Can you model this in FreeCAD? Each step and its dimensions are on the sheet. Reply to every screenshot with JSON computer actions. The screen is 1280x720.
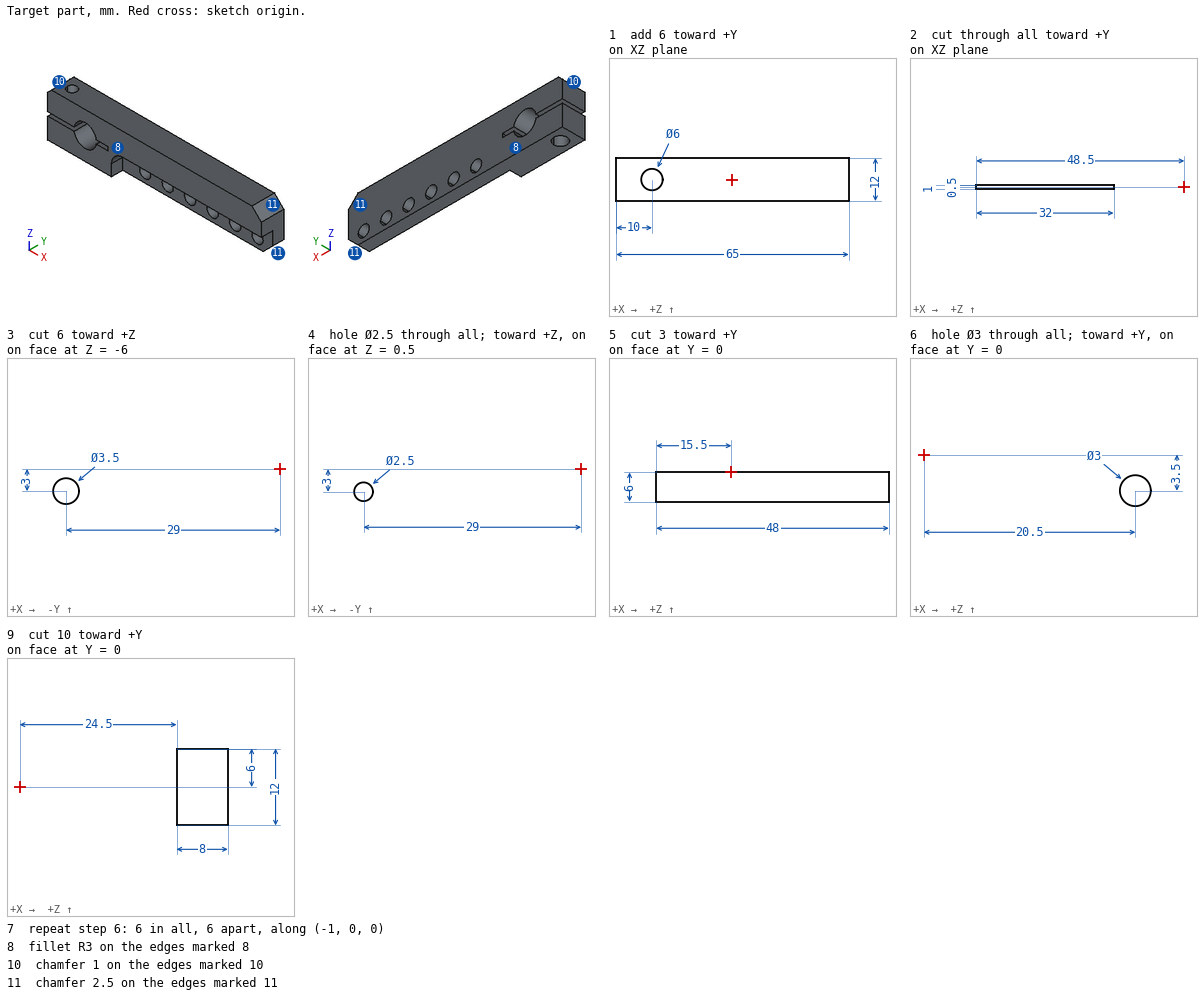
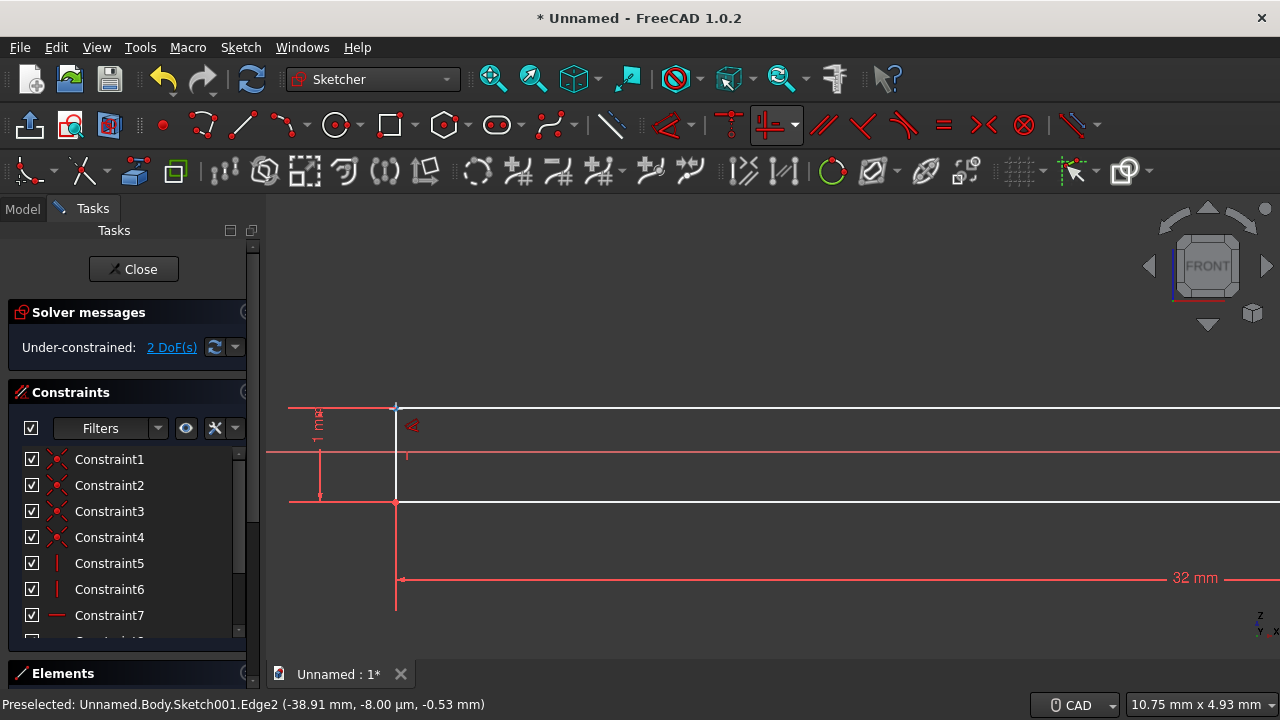
{"action": "left_click", "coordinate": [396, 408]}
{"action": "left_click", "coordinate": [362, 430]}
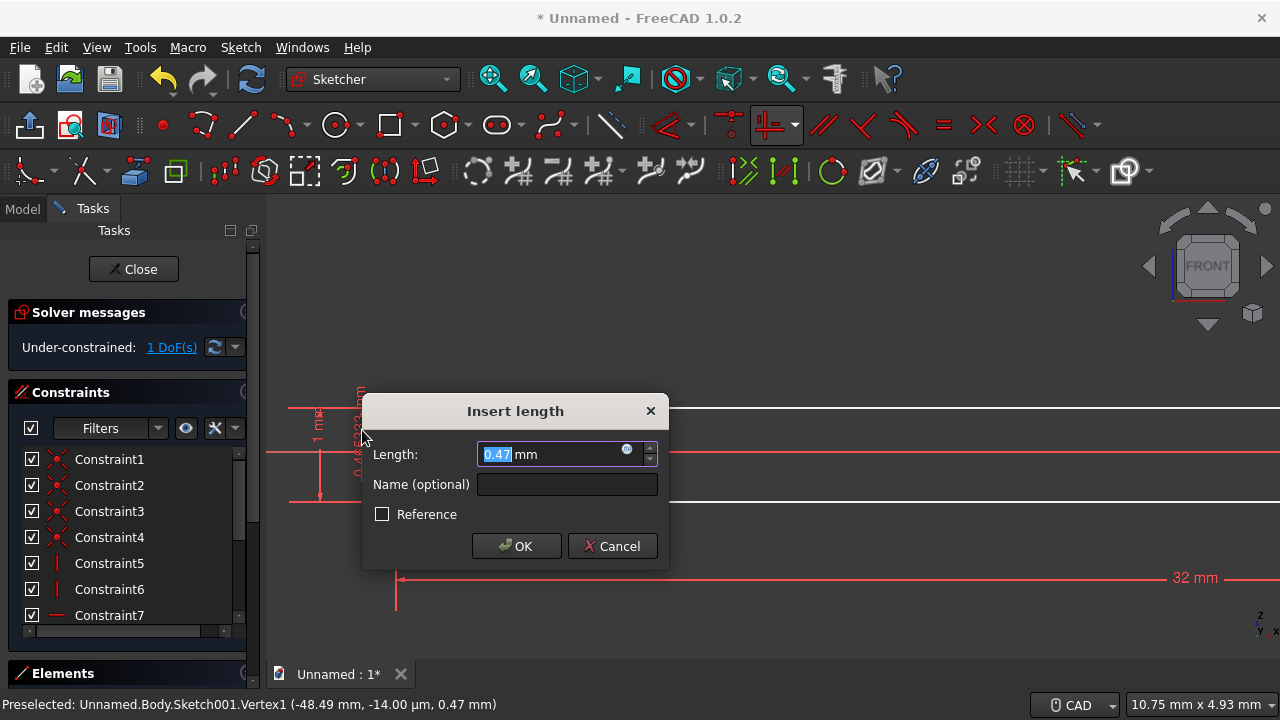
{"action": "type", "text": "0.5"}
{"action": "key", "text": "Return"}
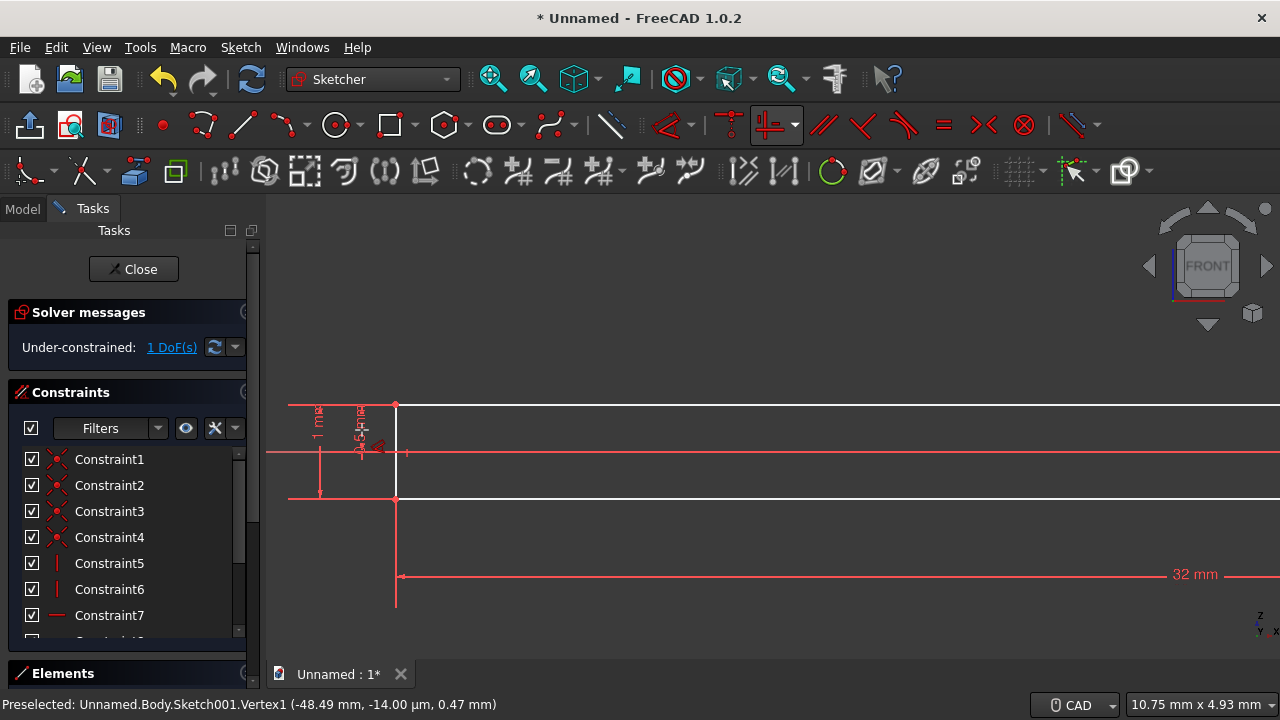
{"action": "scroll", "coordinate": [395, 422], "scroll_direction": "down", "scroll_amount": 10}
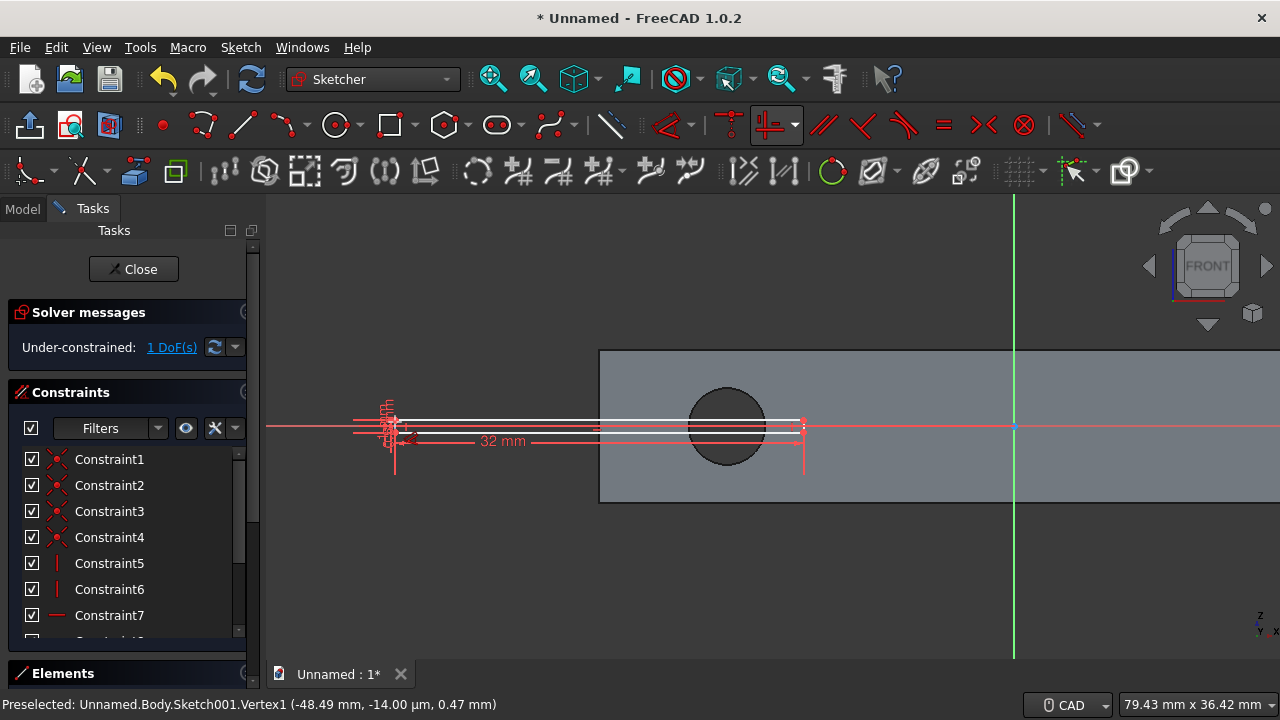
{"action": "left_click", "coordinate": [395, 420]}
{"action": "left_click", "coordinate": [705, 386]}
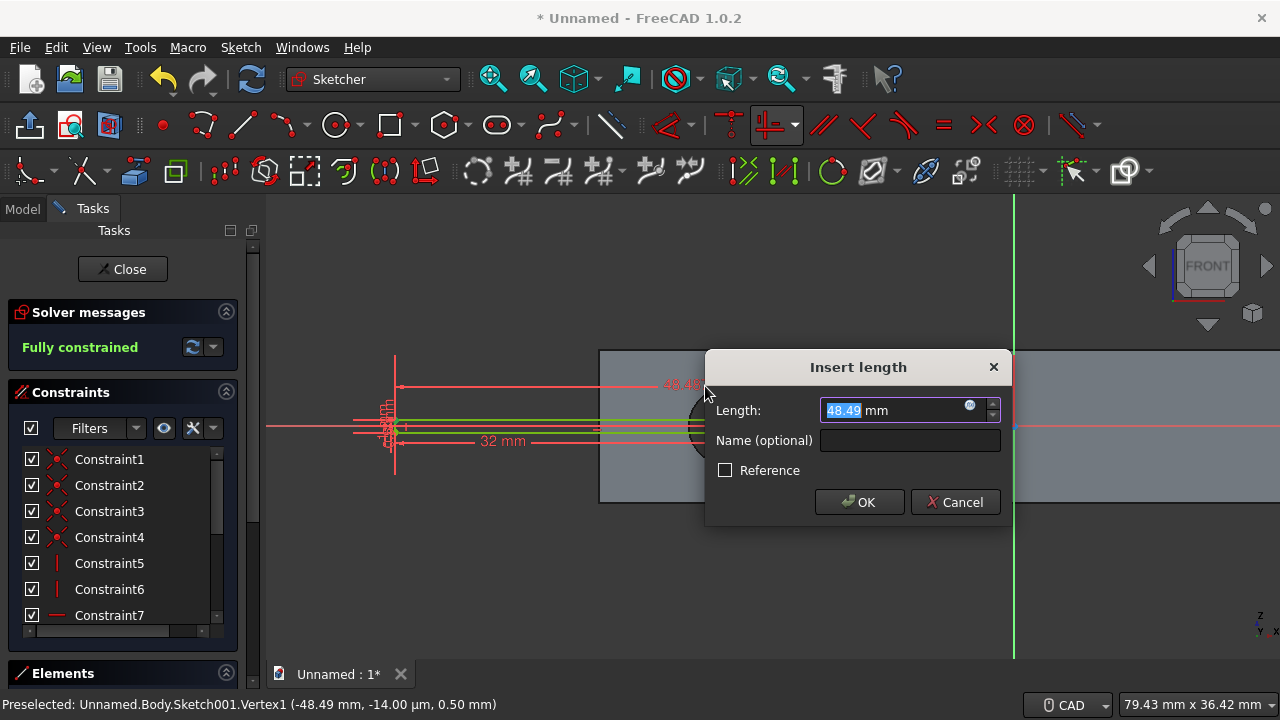
{"action": "type", "text": "48.5"}
{"action": "key", "text": "Return"}
{"action": "key", "text": "Escape"}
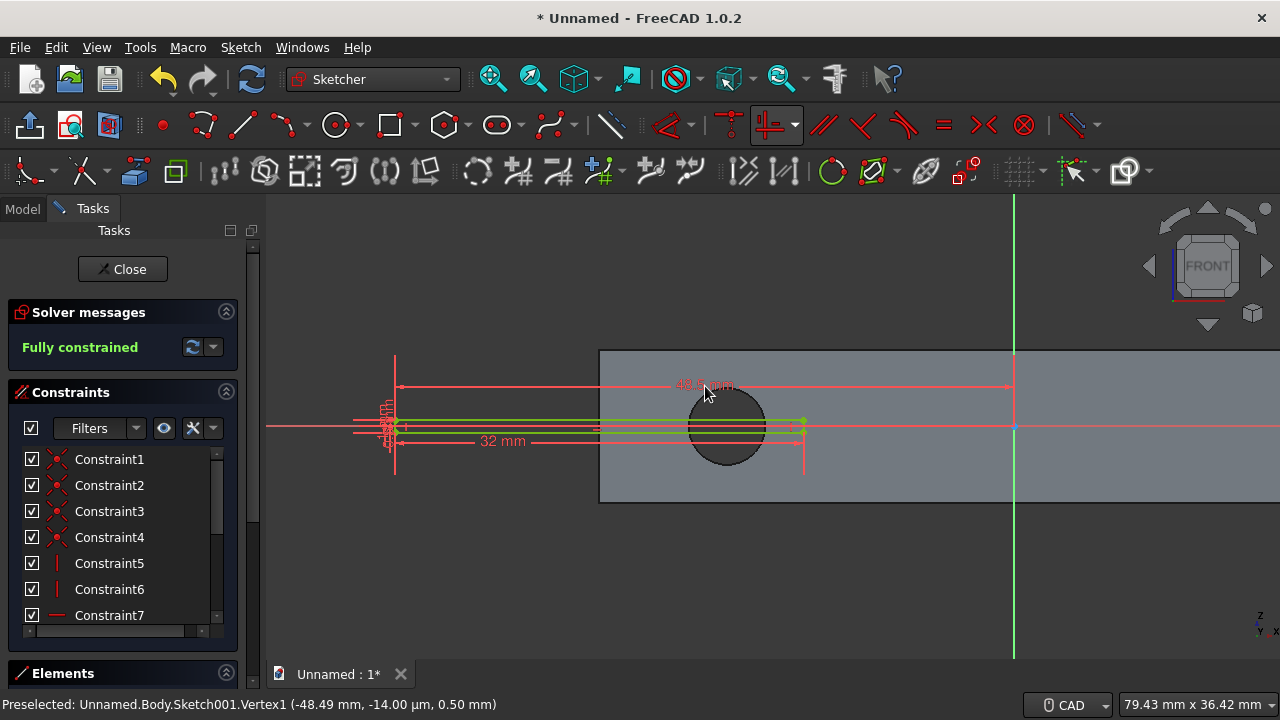
{"action": "left_click", "coordinate": [123, 269]}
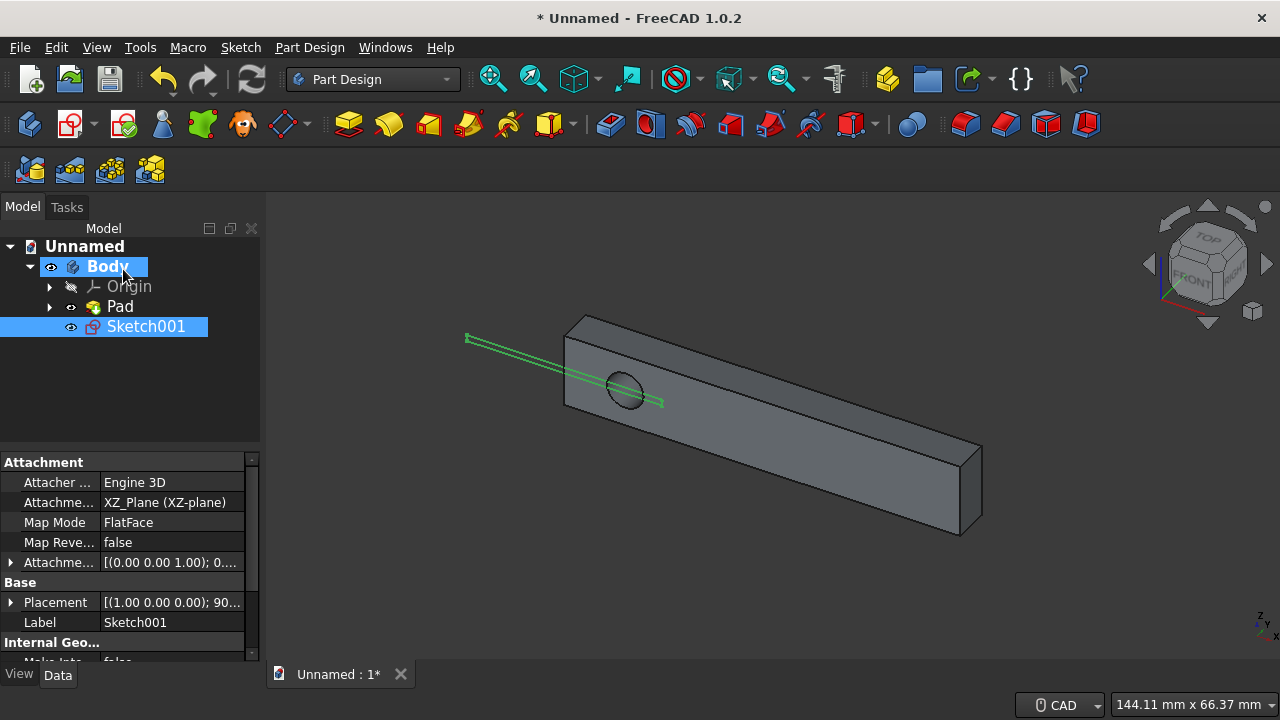
{"action": "left_click", "coordinate": [612, 124]}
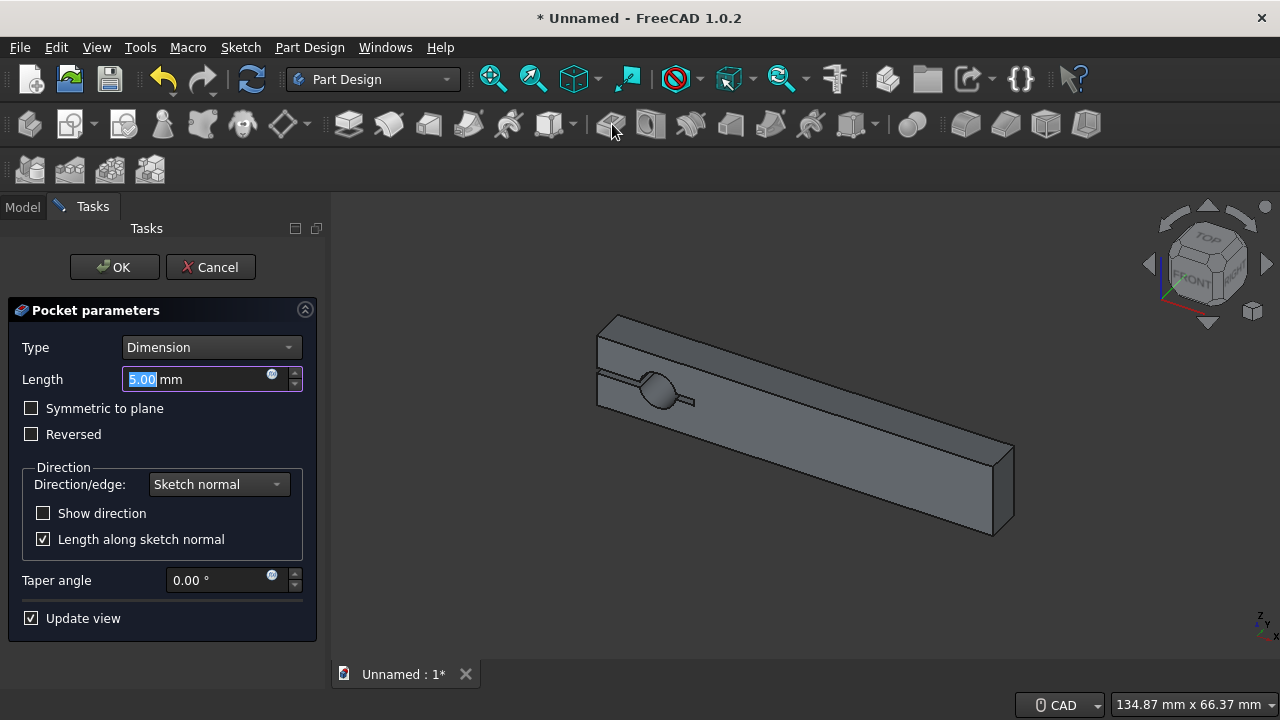
{"action": "left_click", "coordinate": [212, 348]}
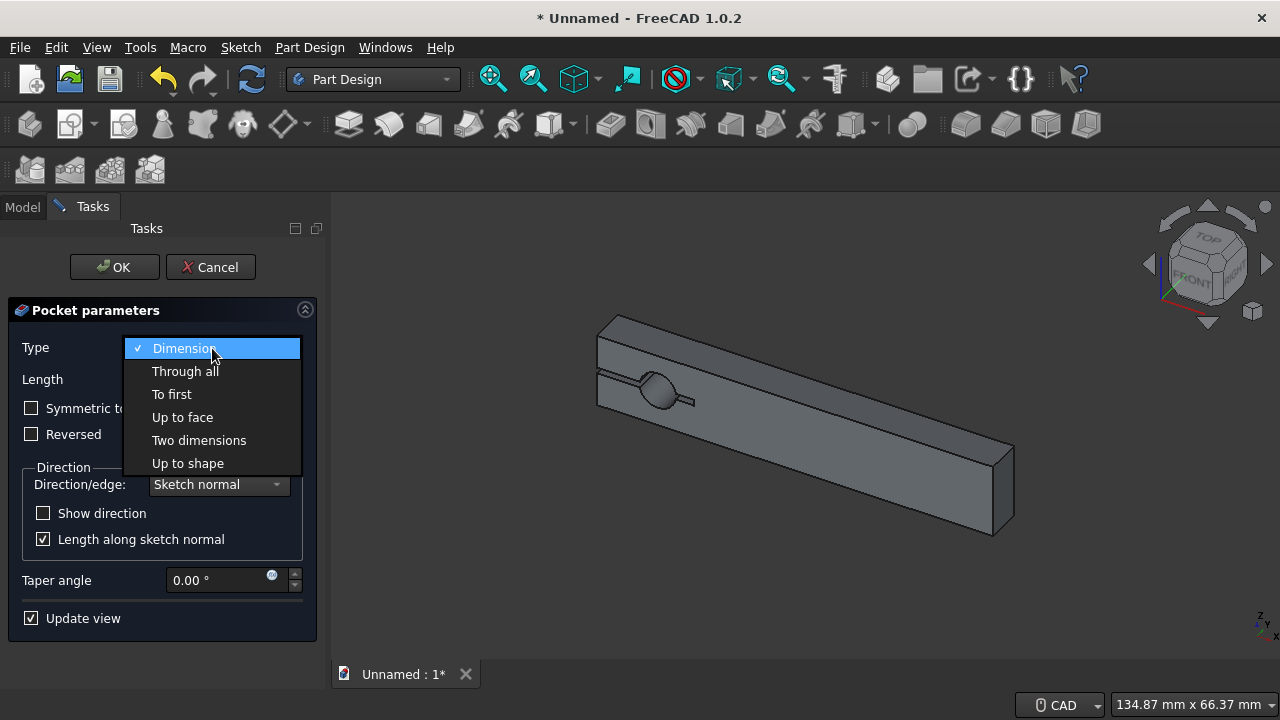
{"action": "left_click", "coordinate": [212, 372]}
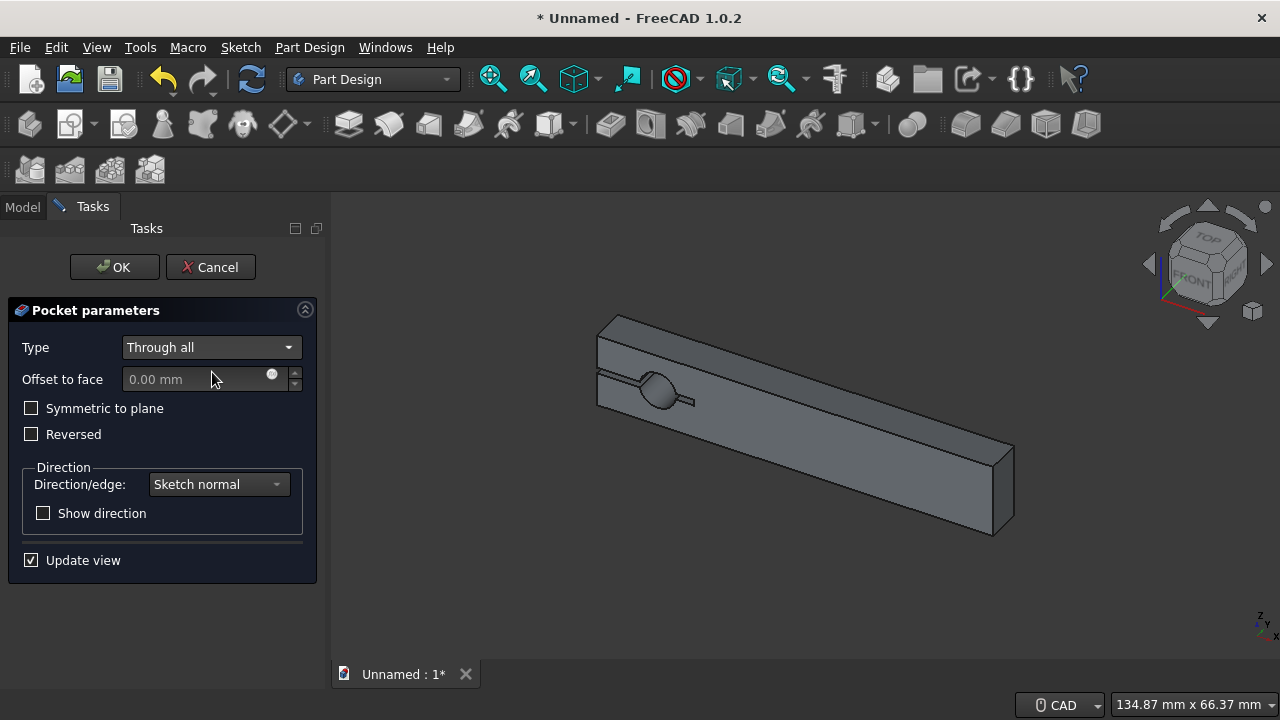
{"action": "left_click", "coordinate": [115, 267]}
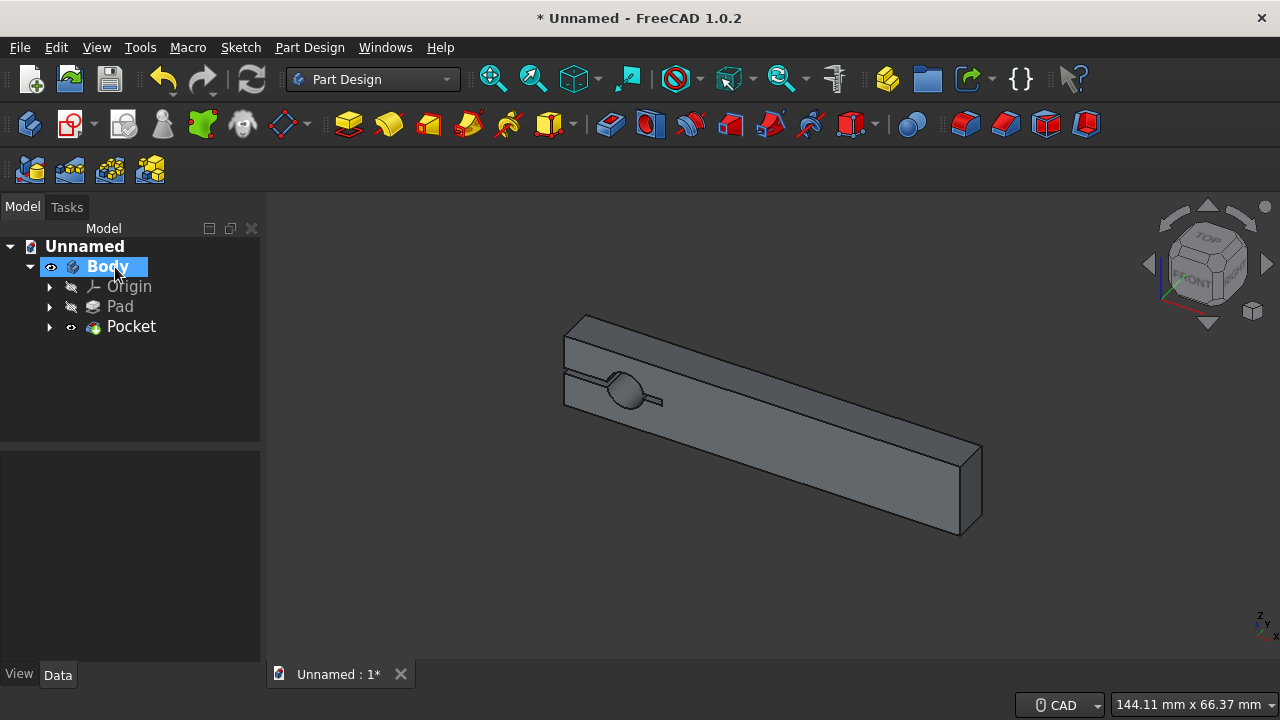
{"action": "key", "text": "5"}